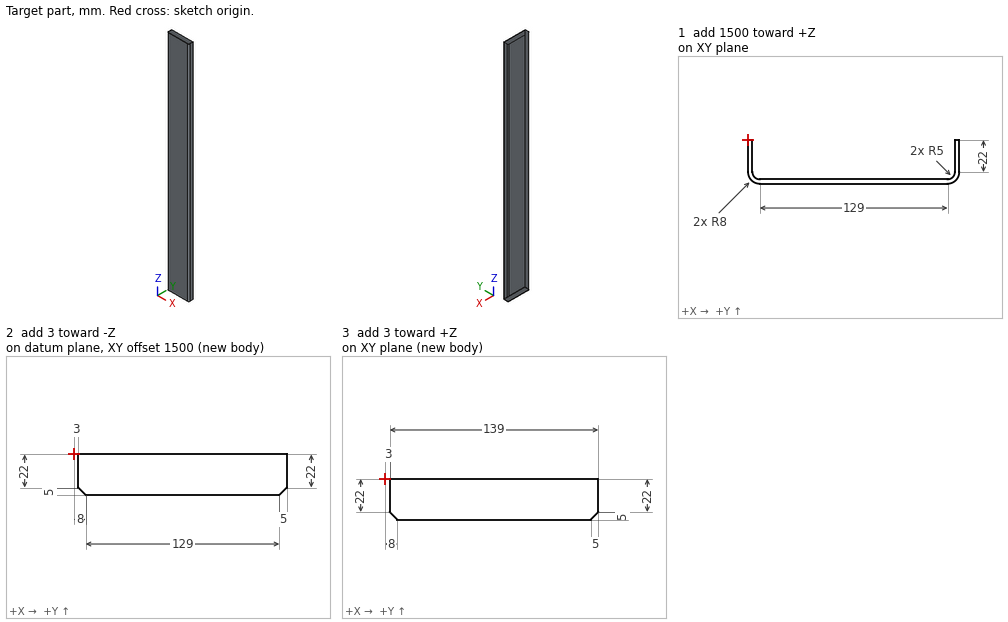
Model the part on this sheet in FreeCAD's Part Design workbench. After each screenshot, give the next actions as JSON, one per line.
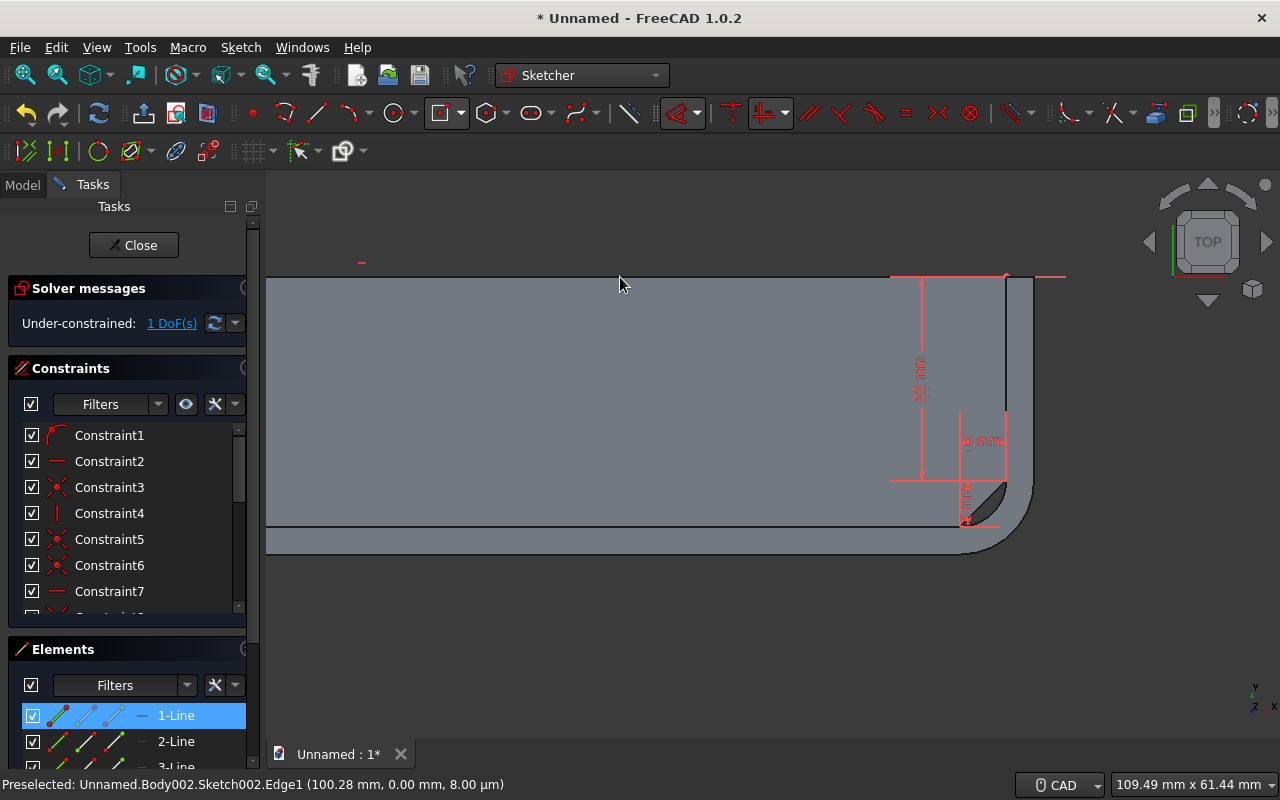
{"action": "key", "text": "l"}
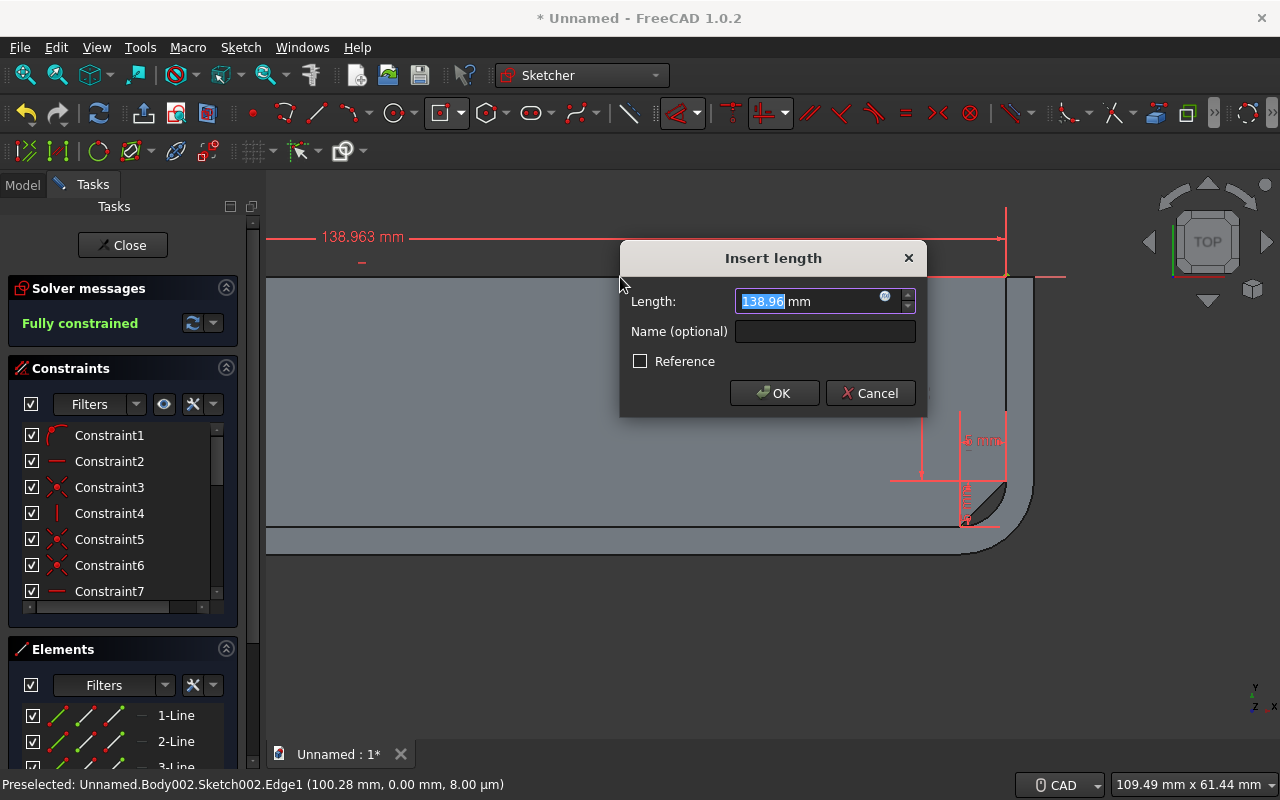
{"action": "type", "text": "139"}
{"action": "key", "text": "Return"}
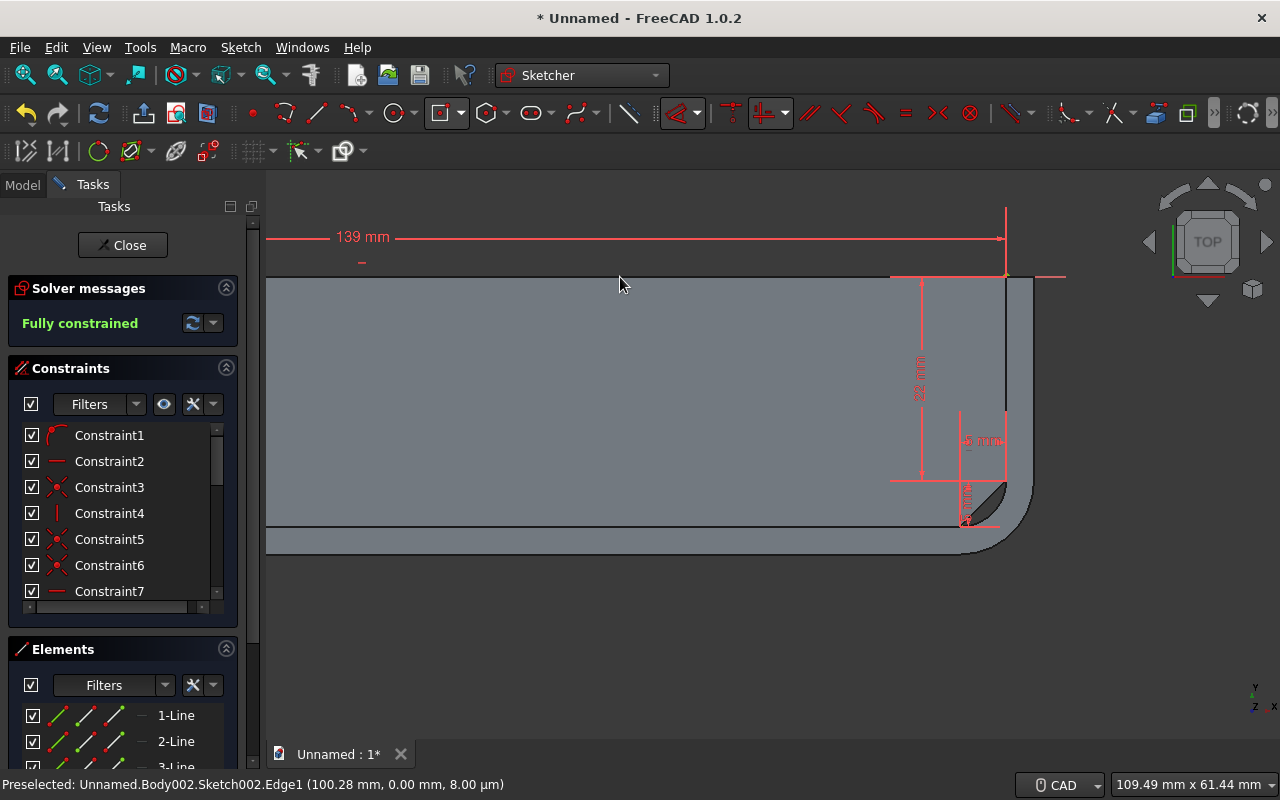
{"action": "left_click", "coordinate": [123, 245]}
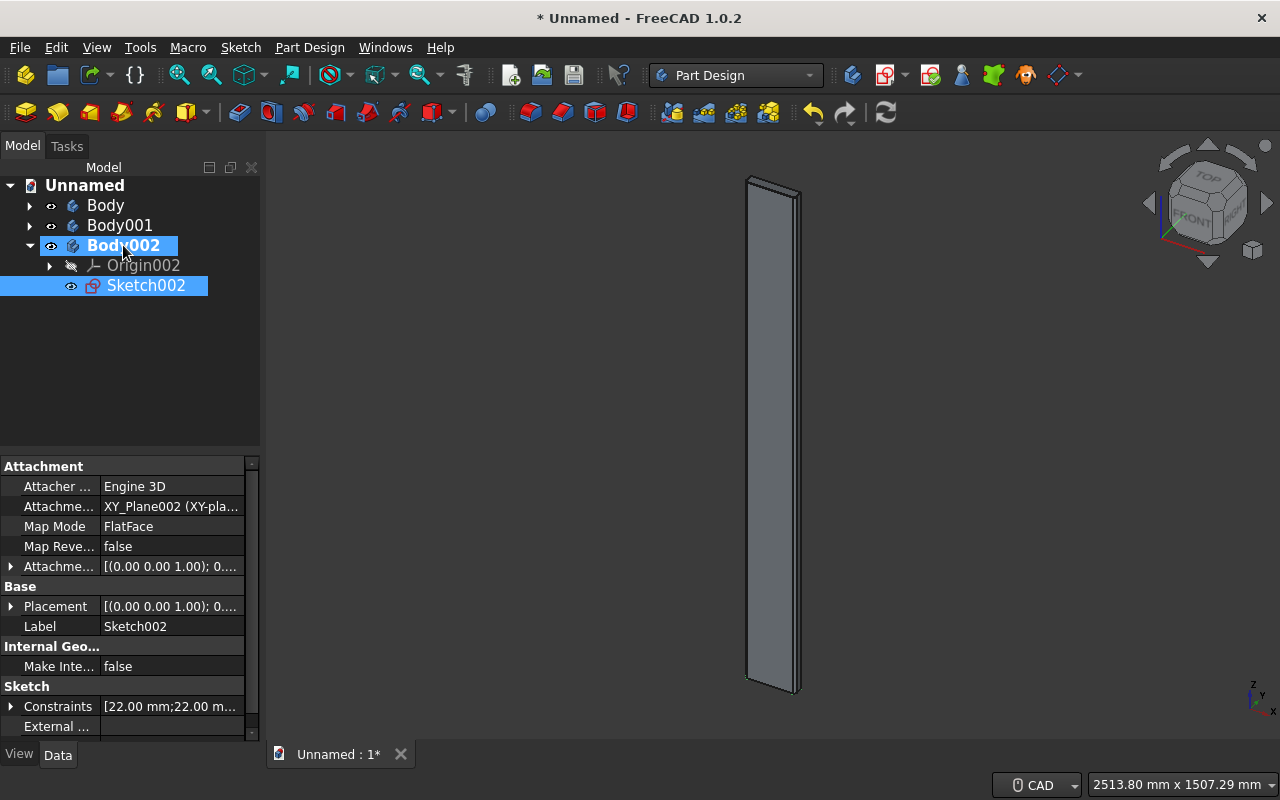
{"action": "left_click", "coordinate": [26, 112]}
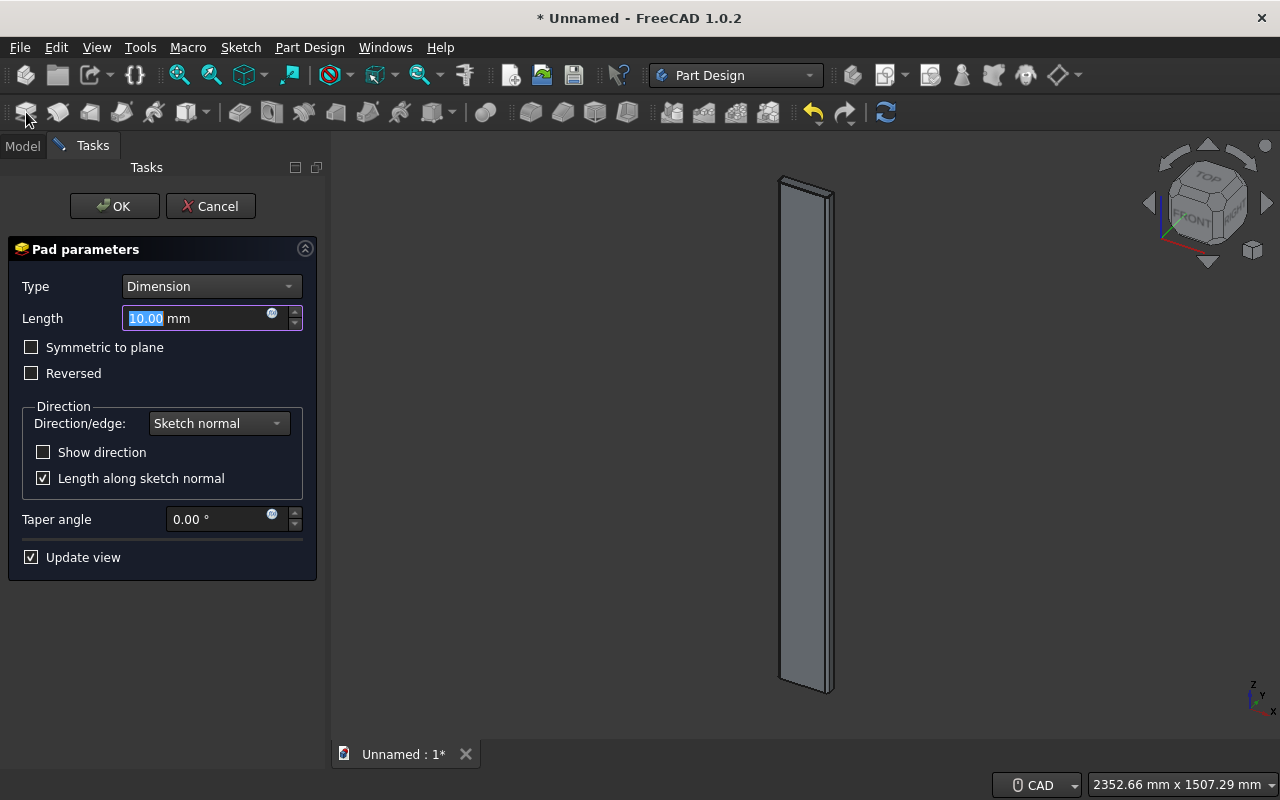
{"action": "type", "text": "3"}
{"action": "key", "text": "Tab"}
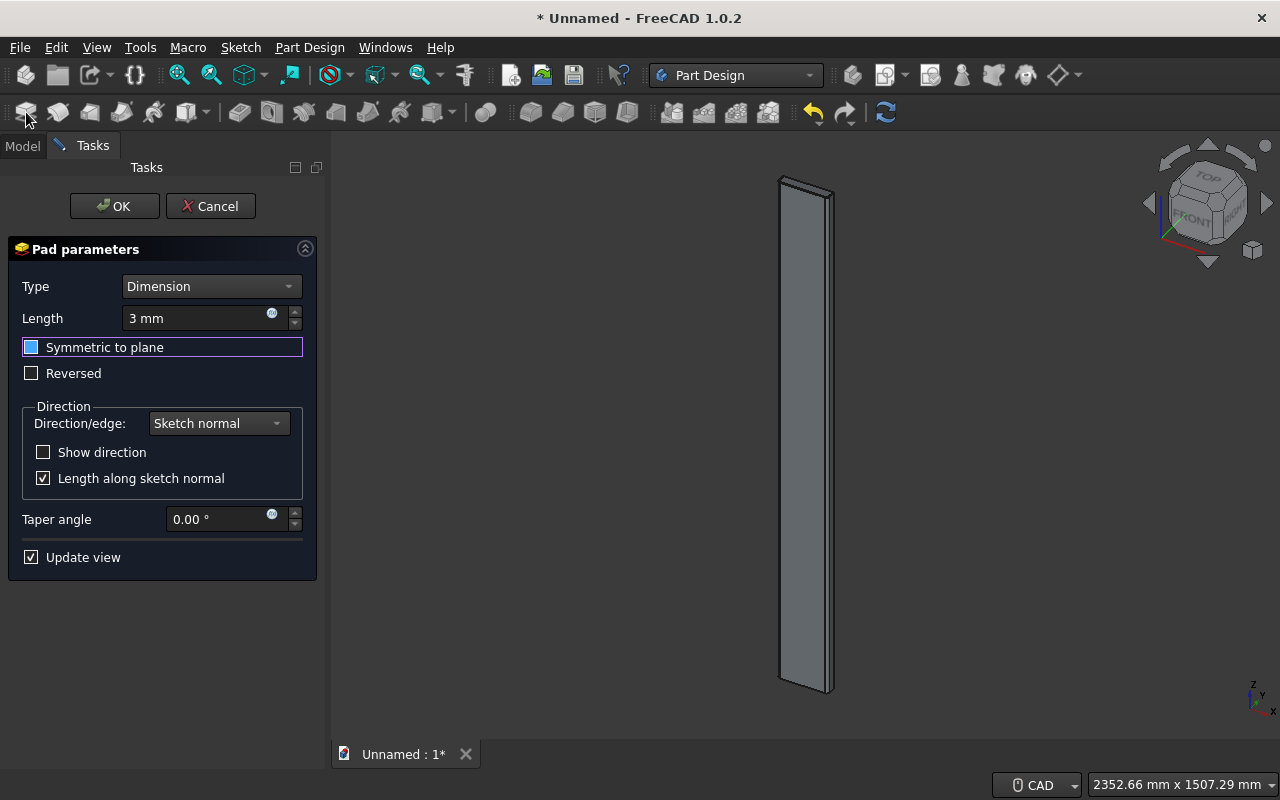
{"action": "left_click", "coordinate": [115, 206]}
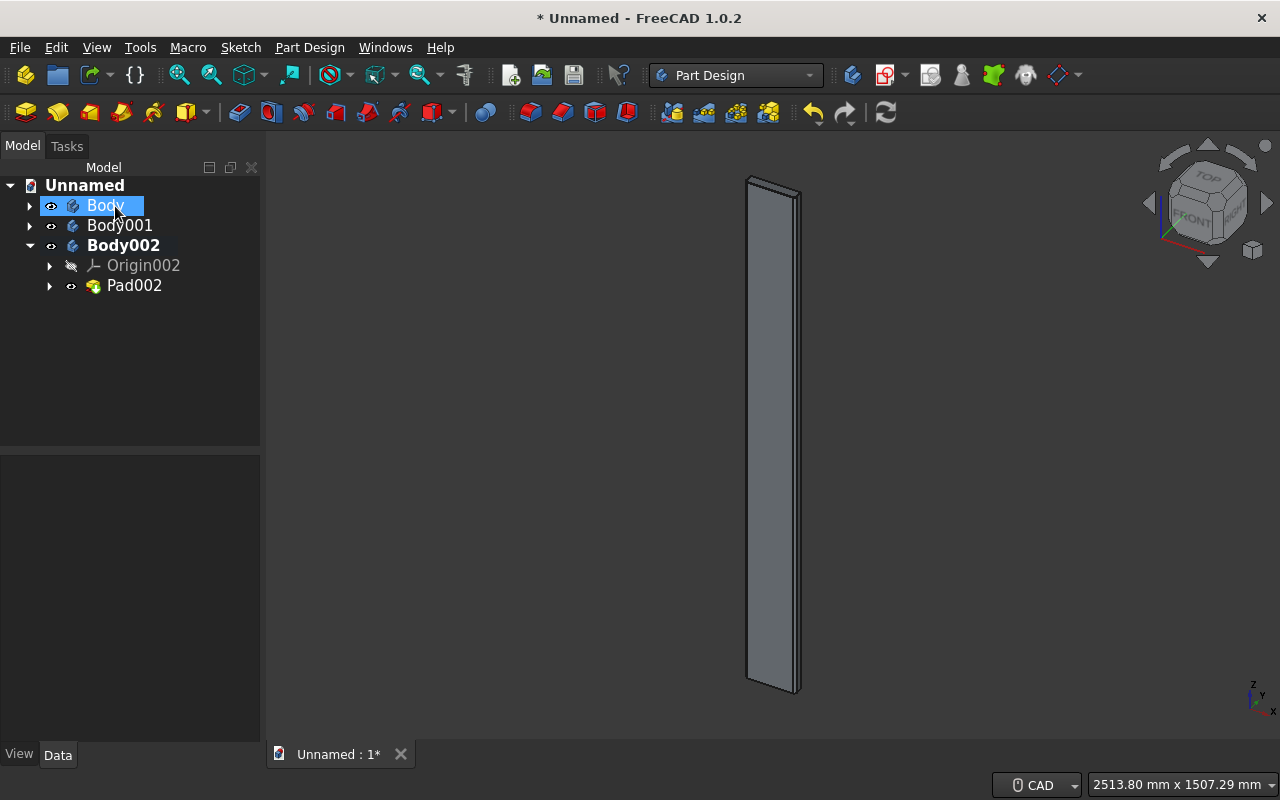
{"action": "key", "text": "0"}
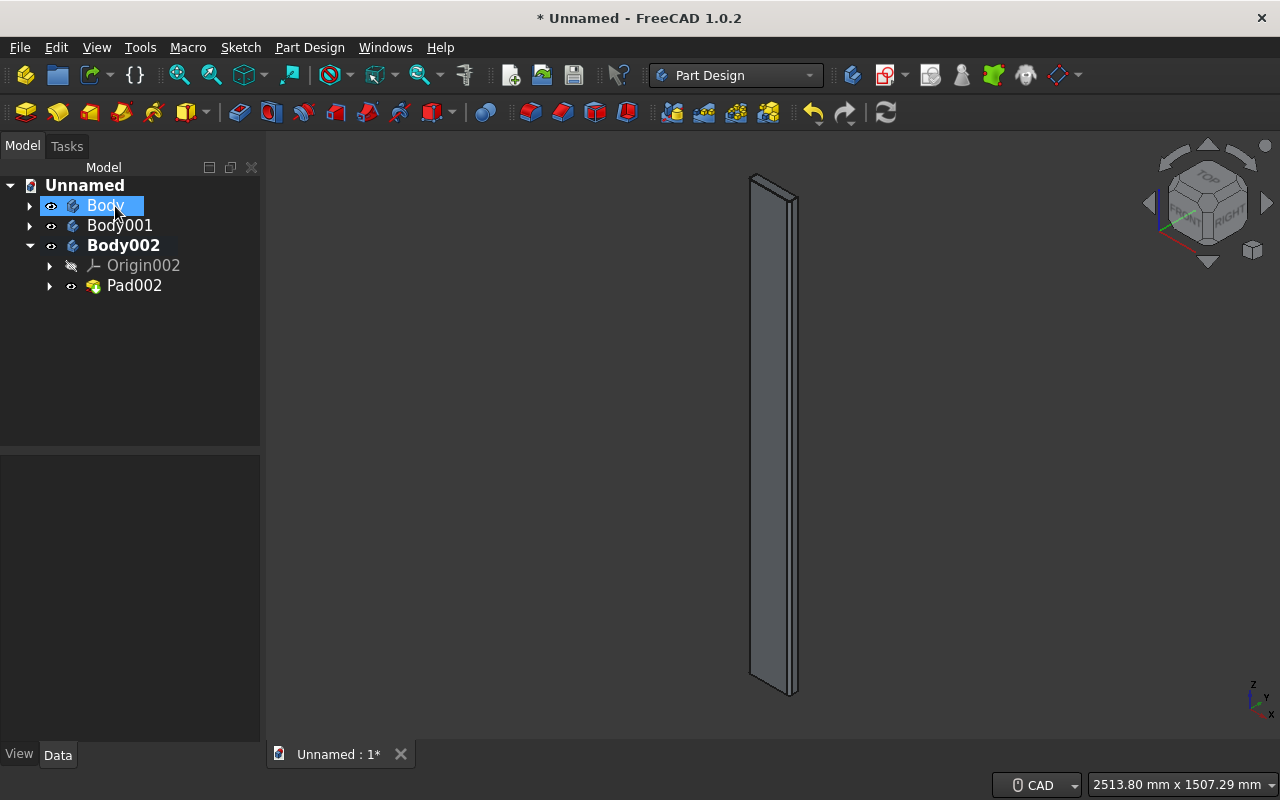
{"action": "left_click", "coordinate": [180, 76]}